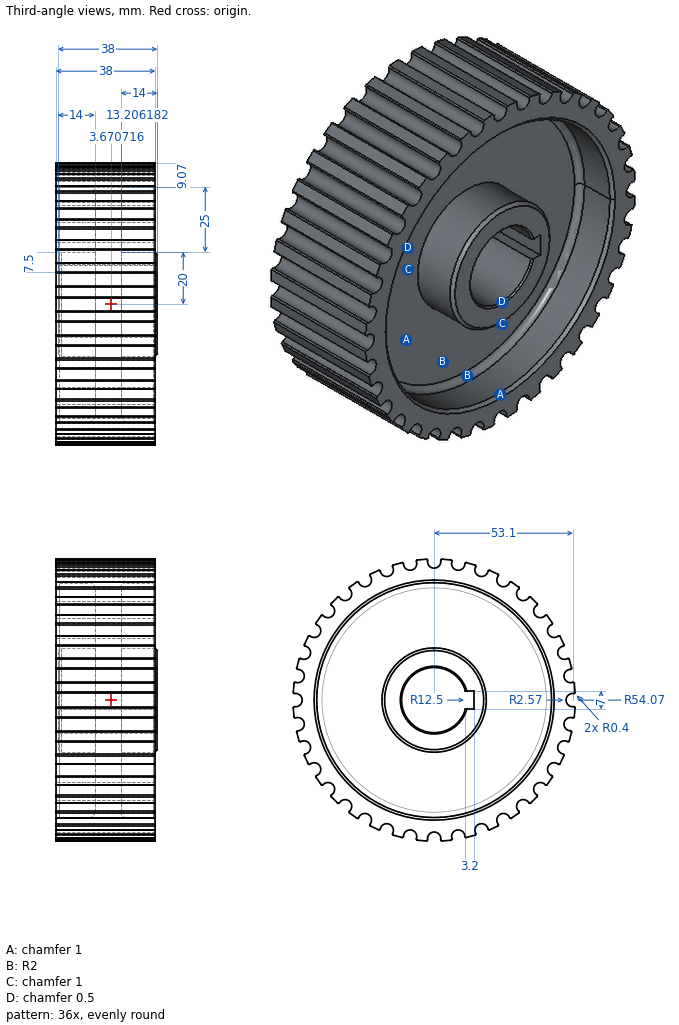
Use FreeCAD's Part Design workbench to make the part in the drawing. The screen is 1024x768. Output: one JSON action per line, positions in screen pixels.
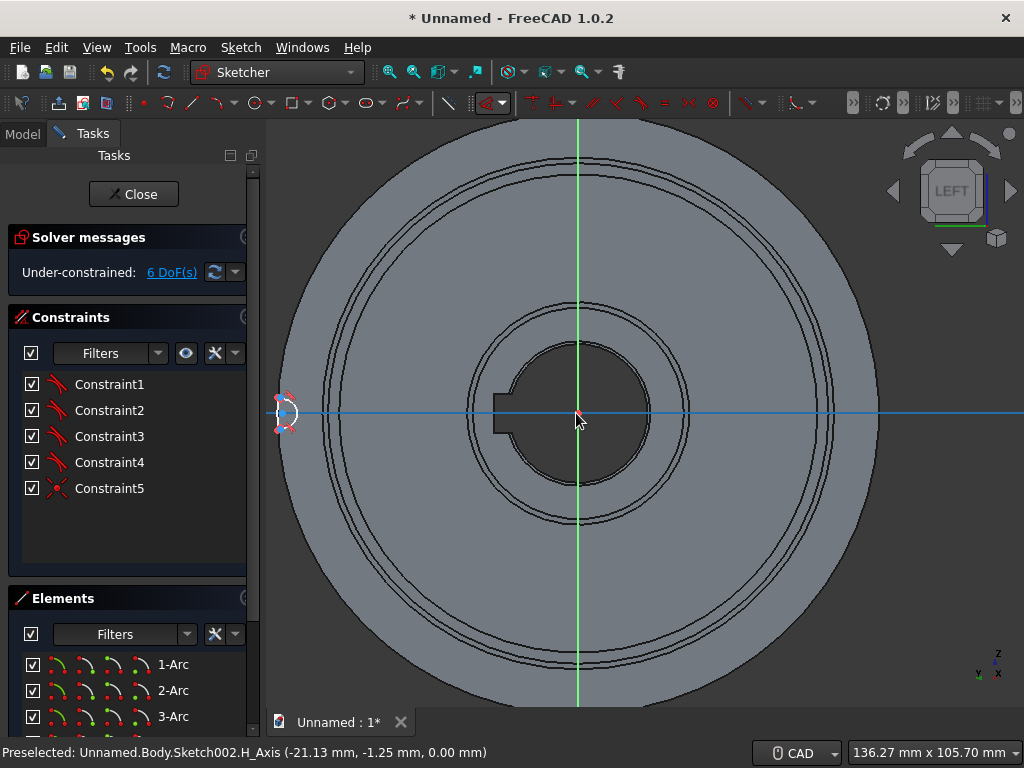
{"action": "scroll", "coordinate": [576, 413], "scroll_direction": "down", "scroll_amount": 5}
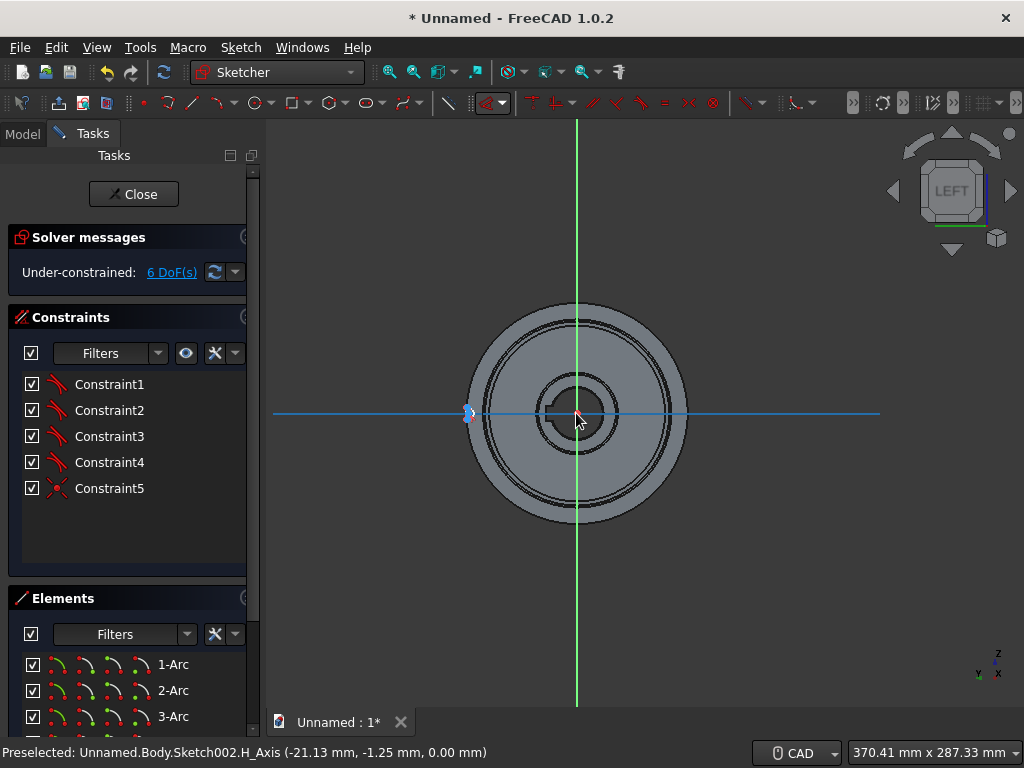
{"action": "scroll", "coordinate": [464, 414], "scroll_direction": "up", "scroll_amount": 15}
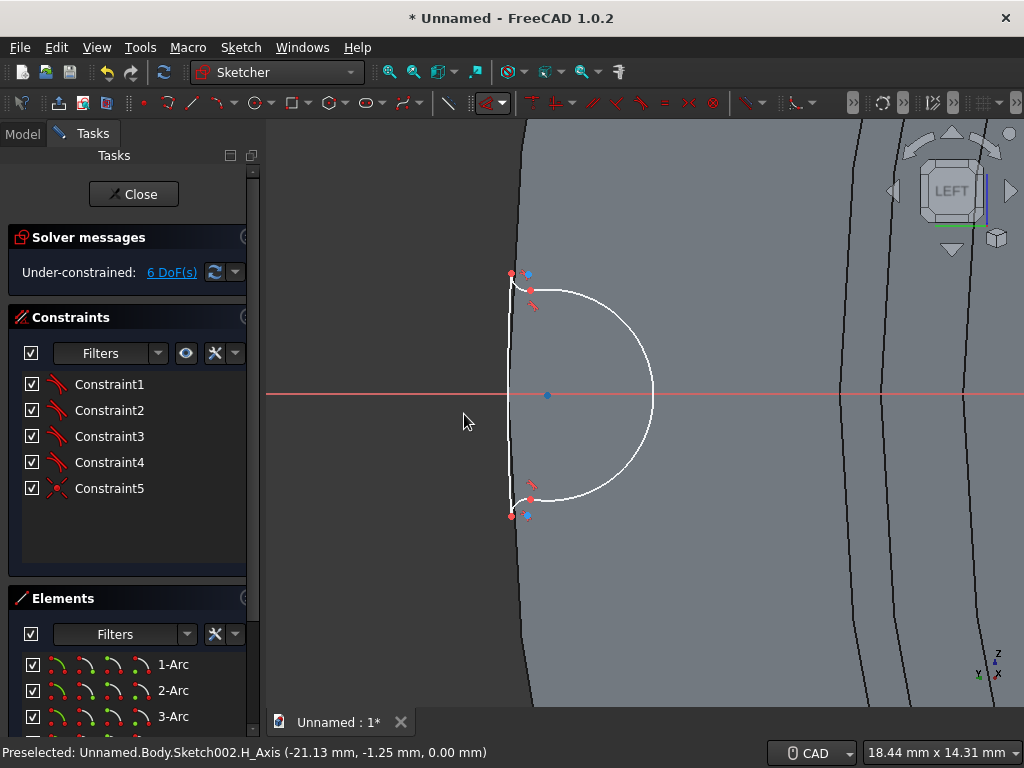
{"action": "scroll", "coordinate": [522, 290], "scroll_direction": "up", "scroll_amount": 3}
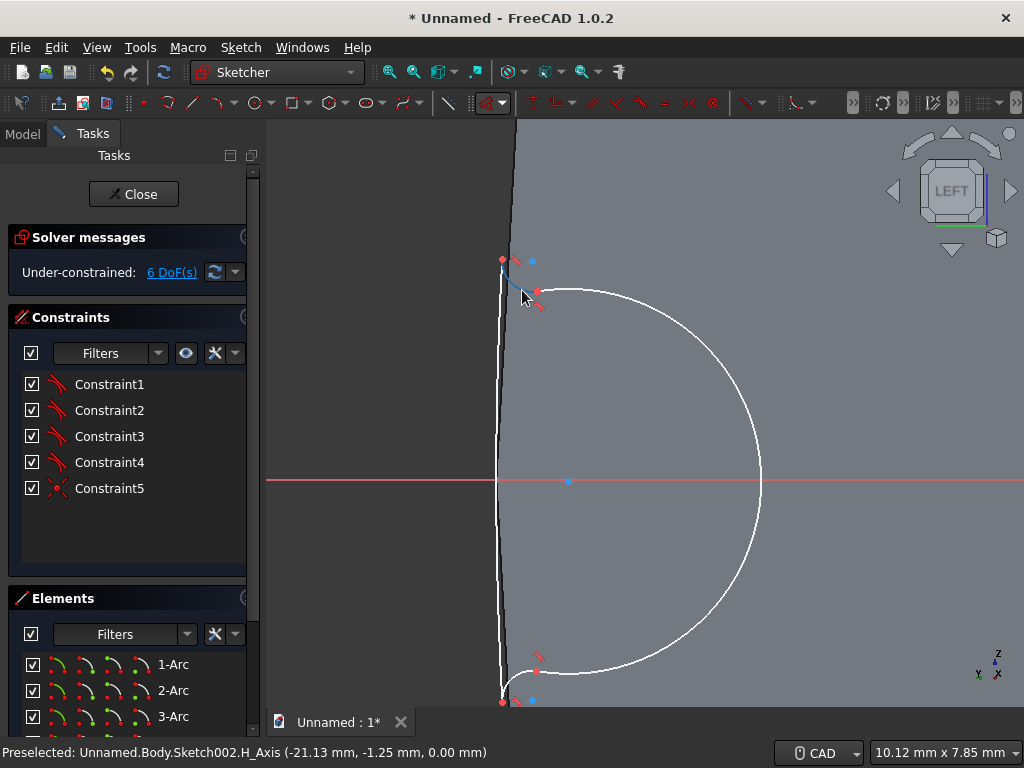
{"action": "left_click", "coordinate": [522, 290]}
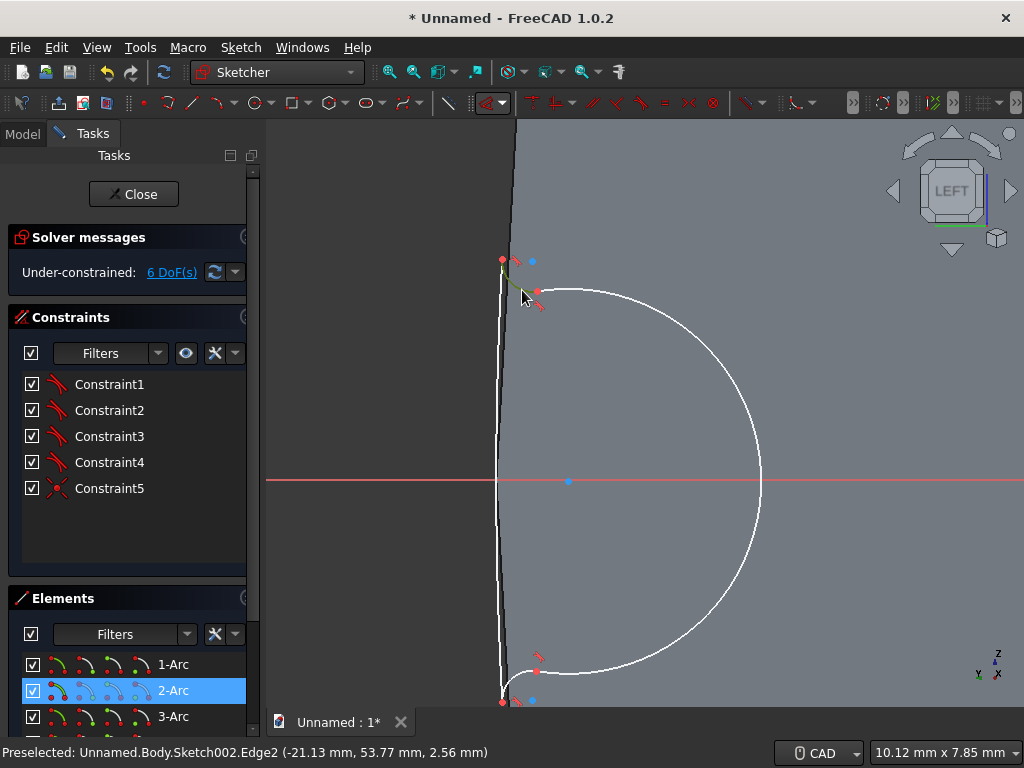
{"action": "left_click", "coordinate": [521, 673]}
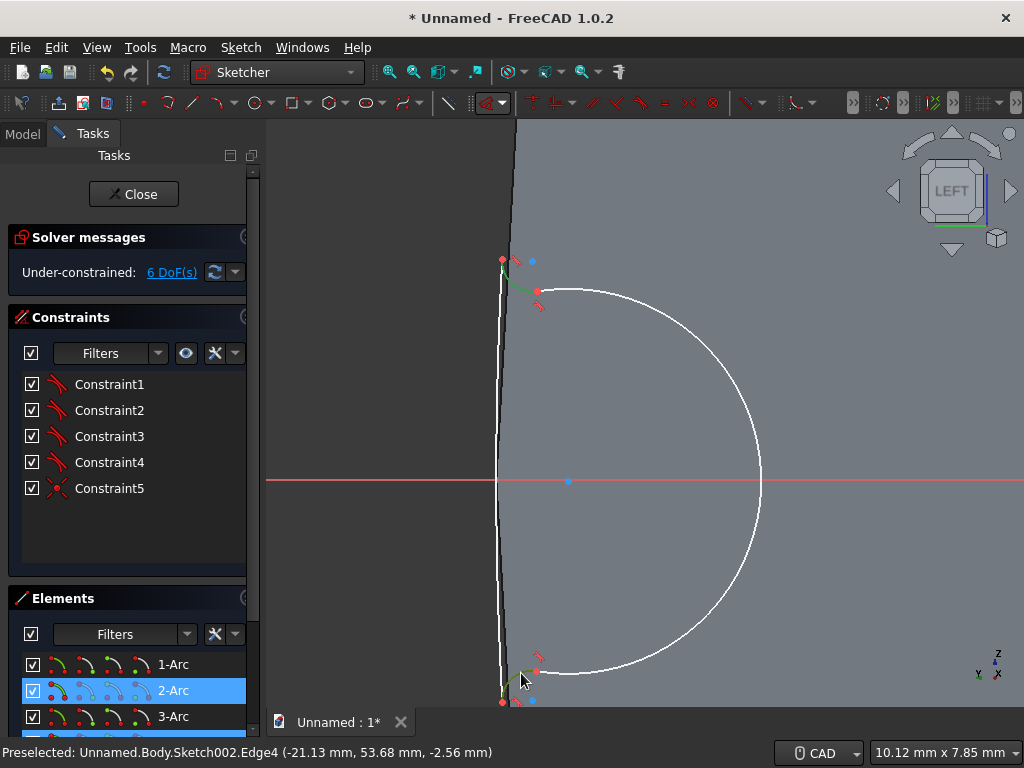
{"action": "left_click", "coordinate": [666, 104]}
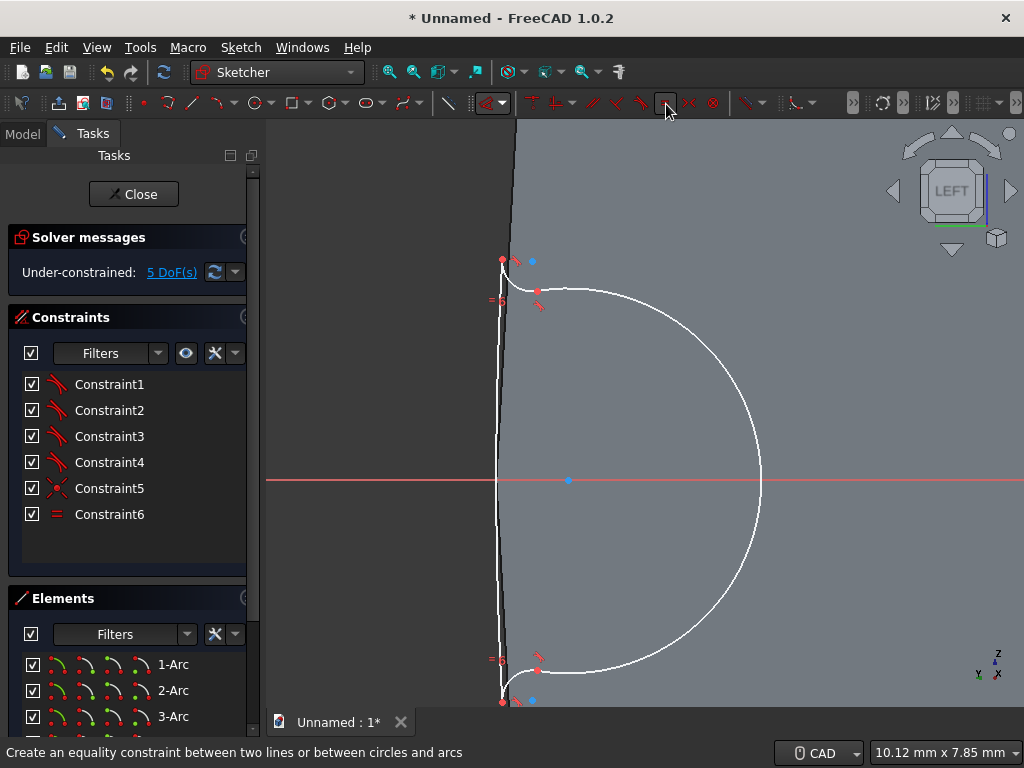
{"action": "left_click", "coordinate": [569, 481]}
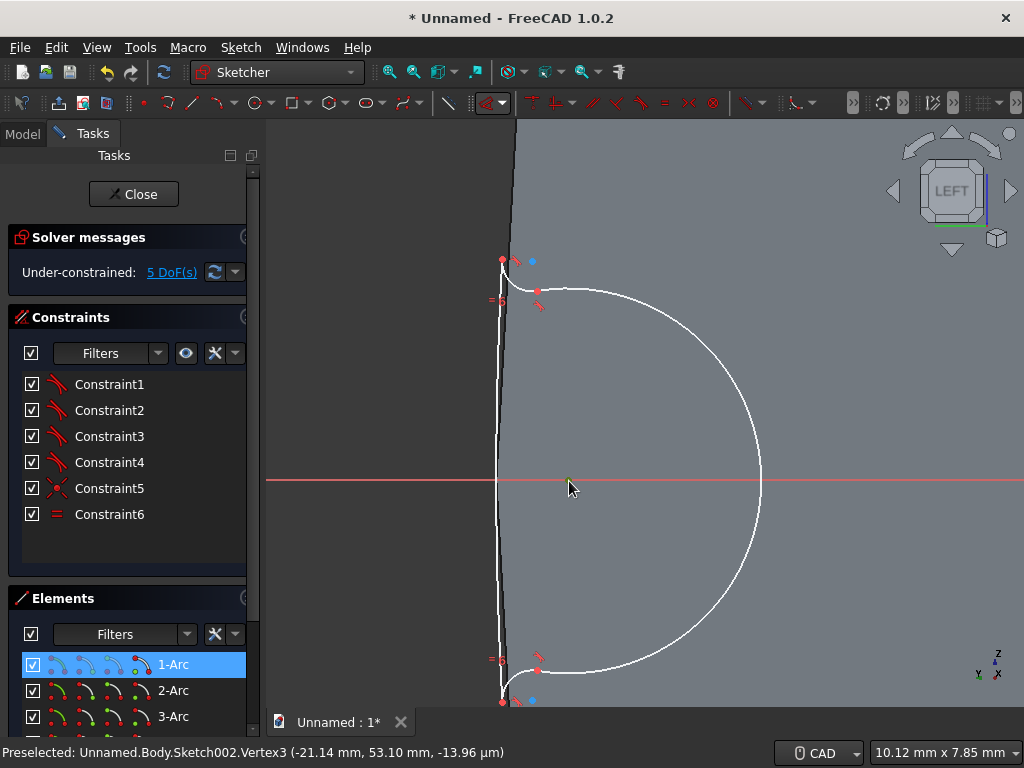
{"action": "left_click", "coordinate": [334, 480]}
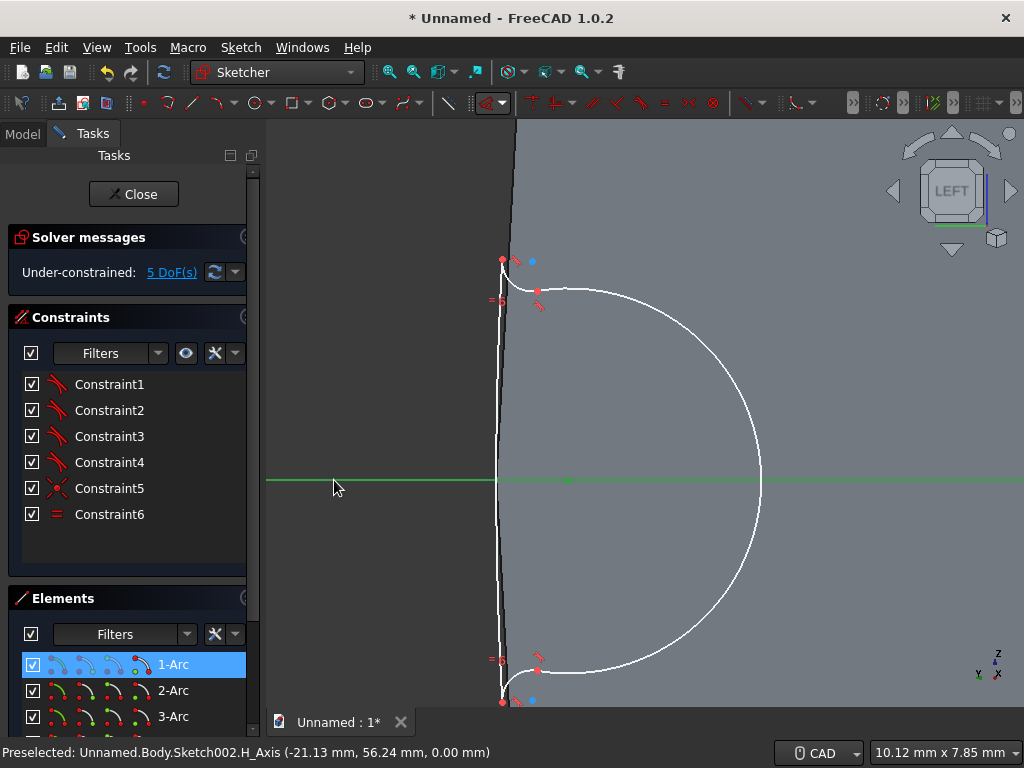
{"action": "left_click", "coordinate": [532, 104]}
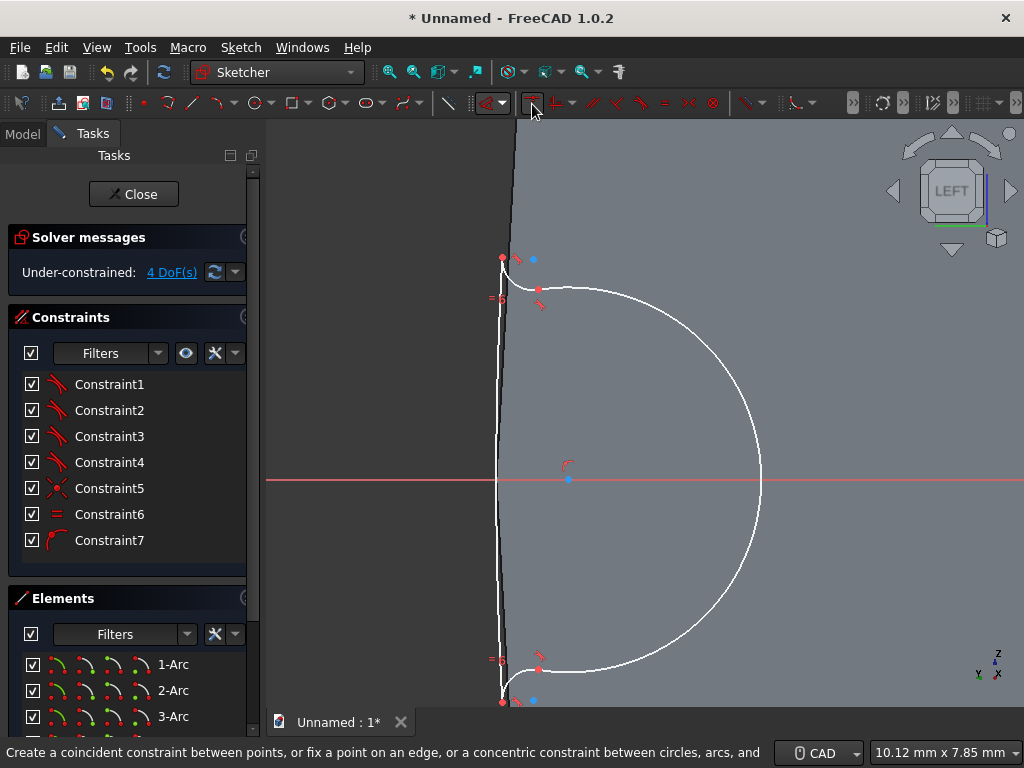
{"action": "left_click", "coordinate": [717, 603]}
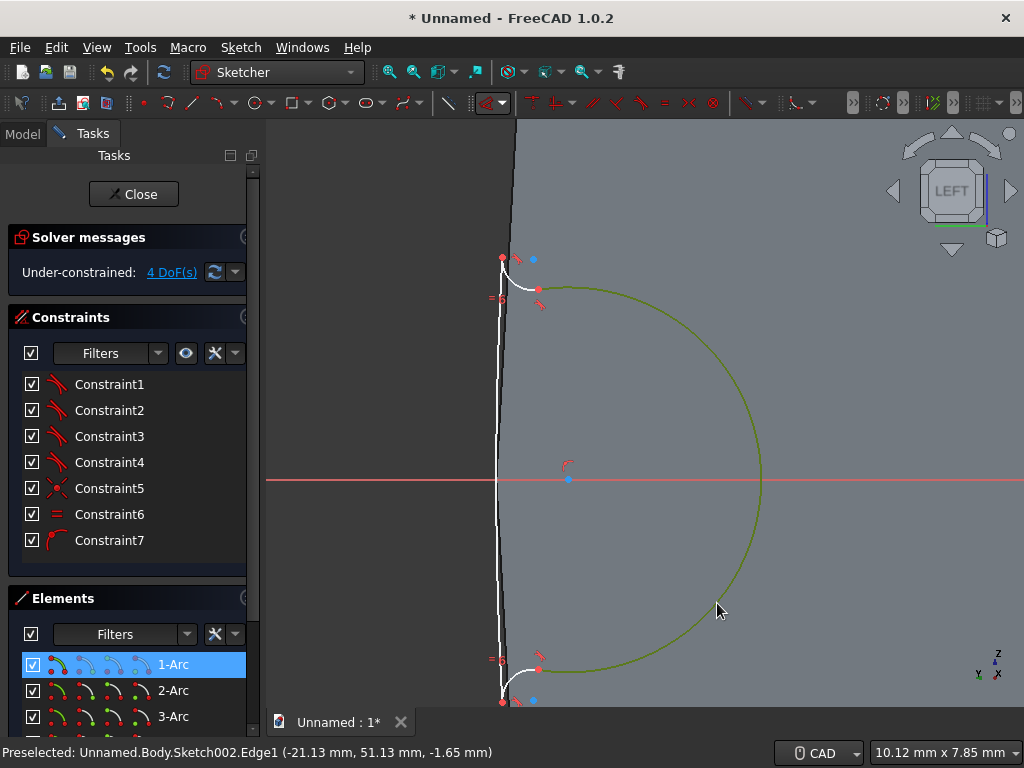
{"action": "key", "text": "k r"}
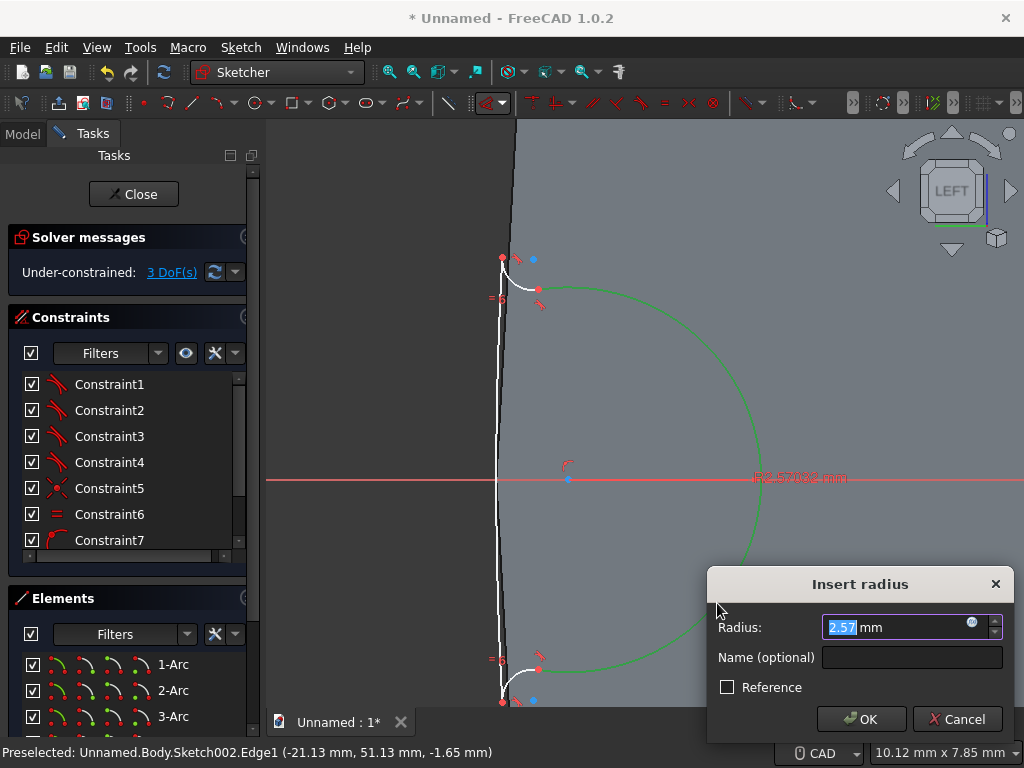
{"action": "type", "text": "2.57"}
{"action": "key", "text": "Return"}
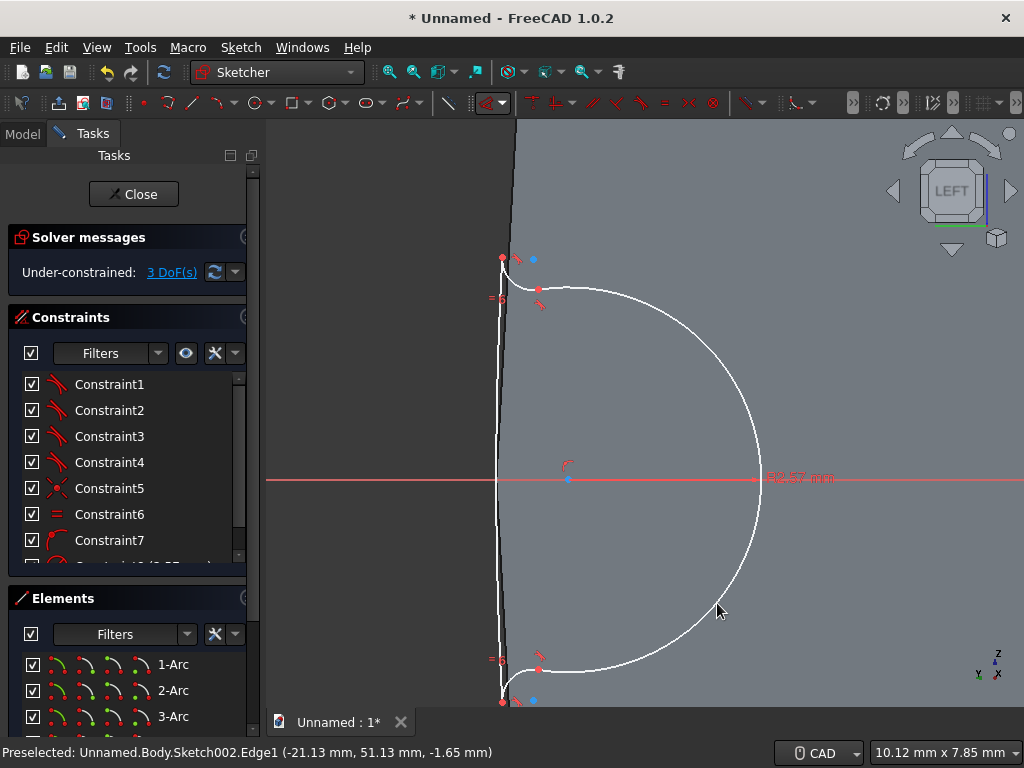
{"action": "scroll", "coordinate": [522, 288], "scroll_direction": "up", "scroll_amount": 2}